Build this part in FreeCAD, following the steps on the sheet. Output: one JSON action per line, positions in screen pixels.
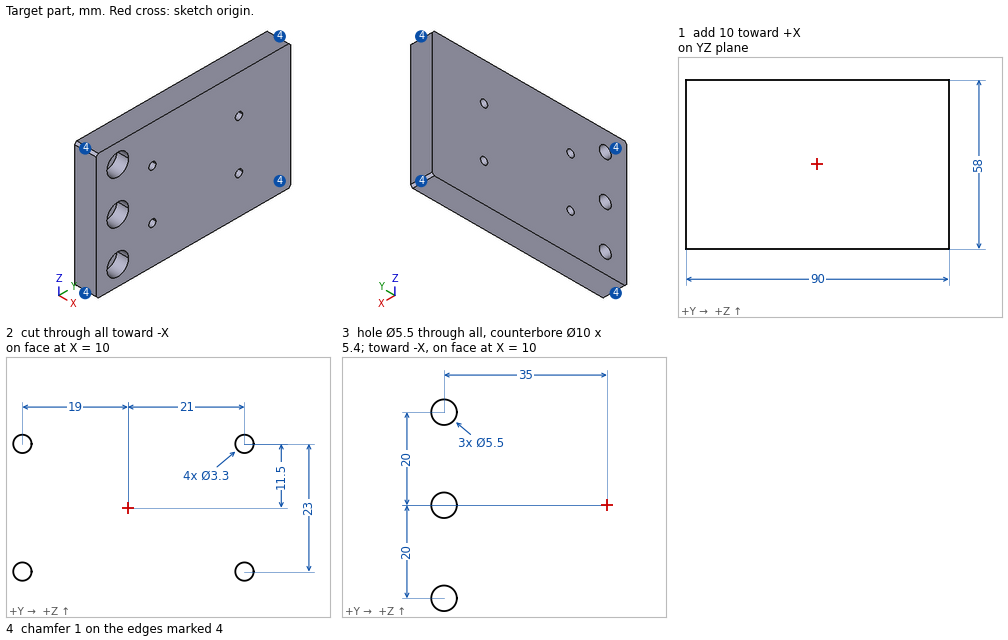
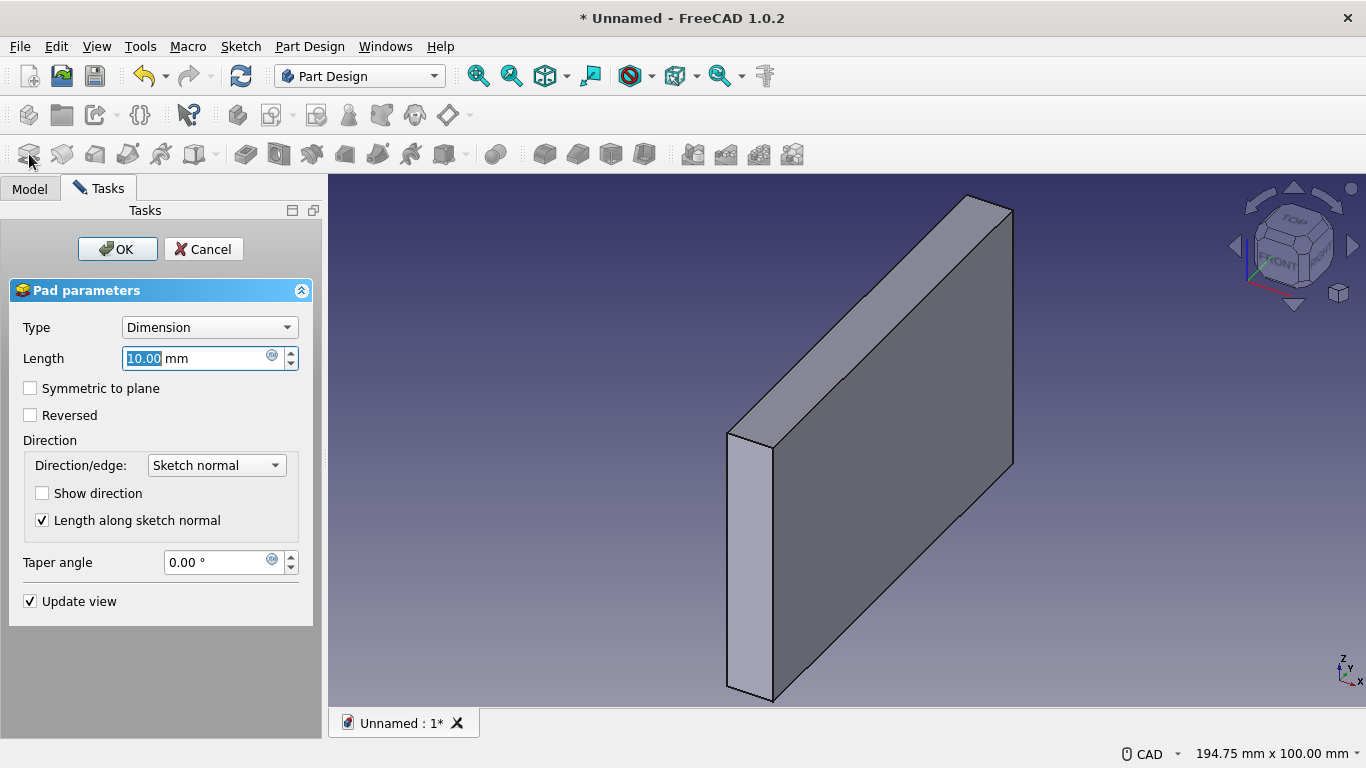
{"action": "type", "text": "10"}
{"action": "key", "text": "Tab"}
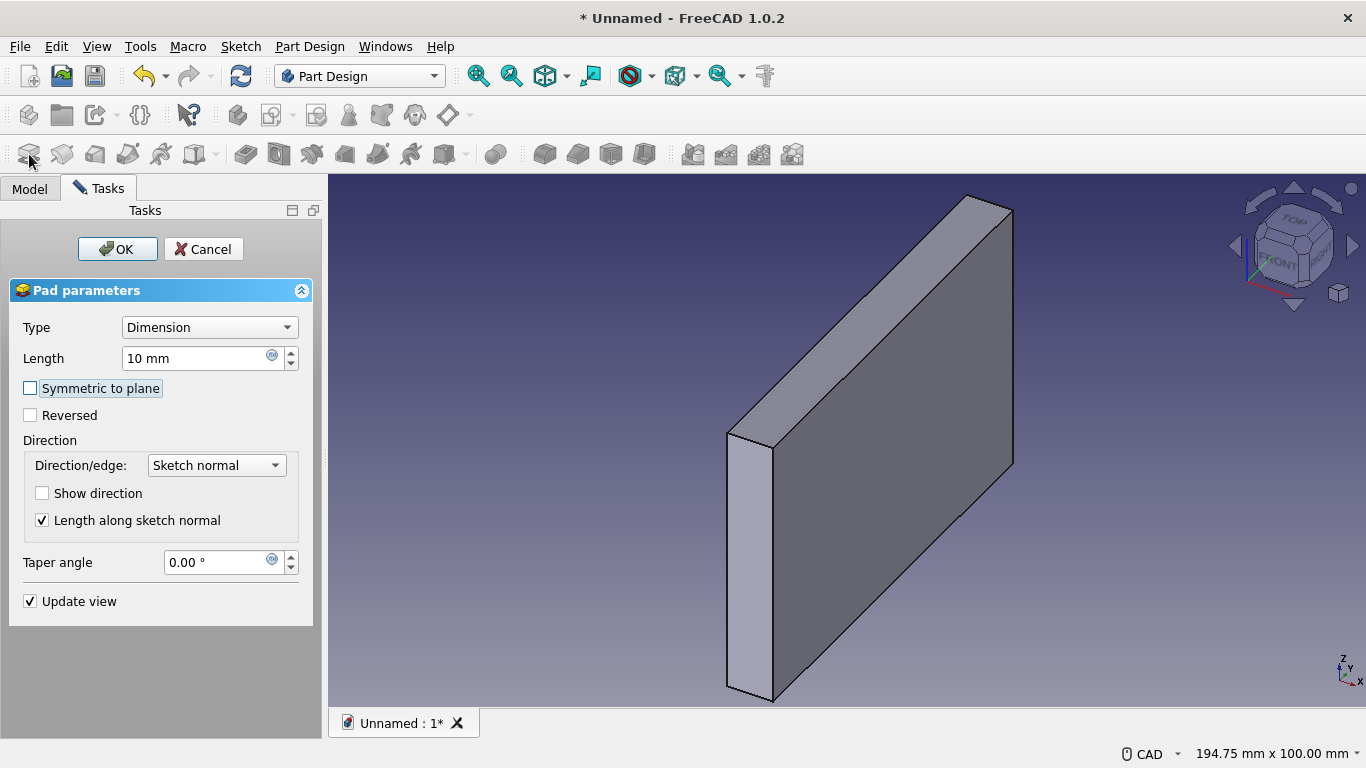
{"action": "left_click", "coordinate": [118, 249]}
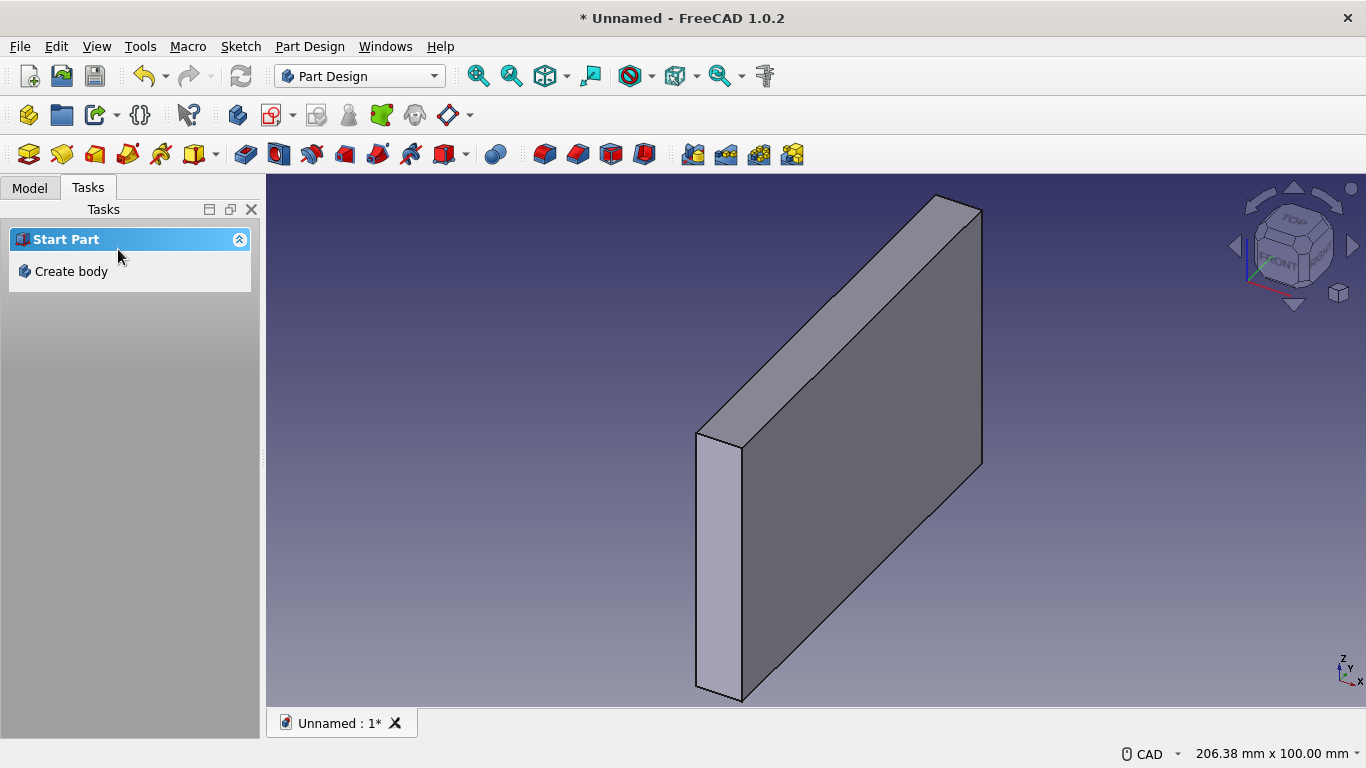
{"action": "left_click", "coordinate": [896, 421]}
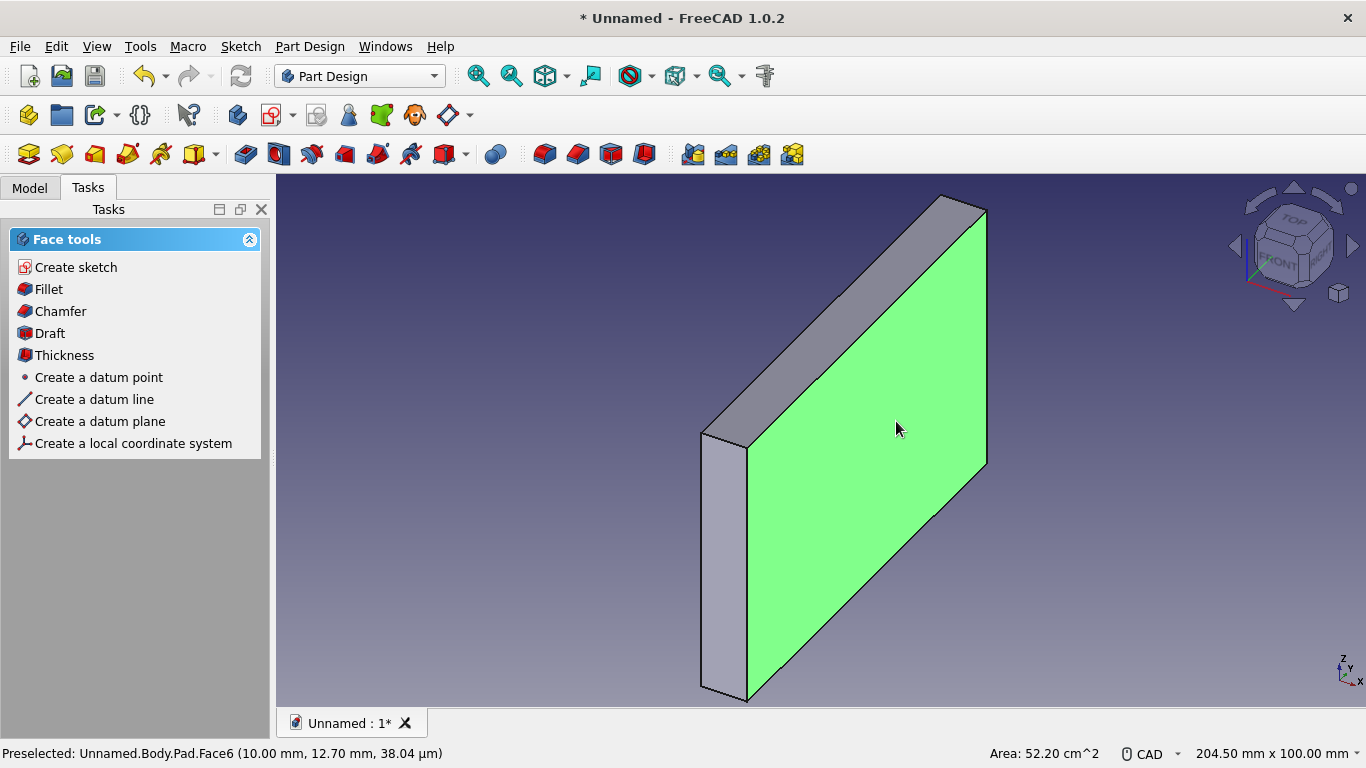
{"action": "left_click", "coordinate": [270, 116]}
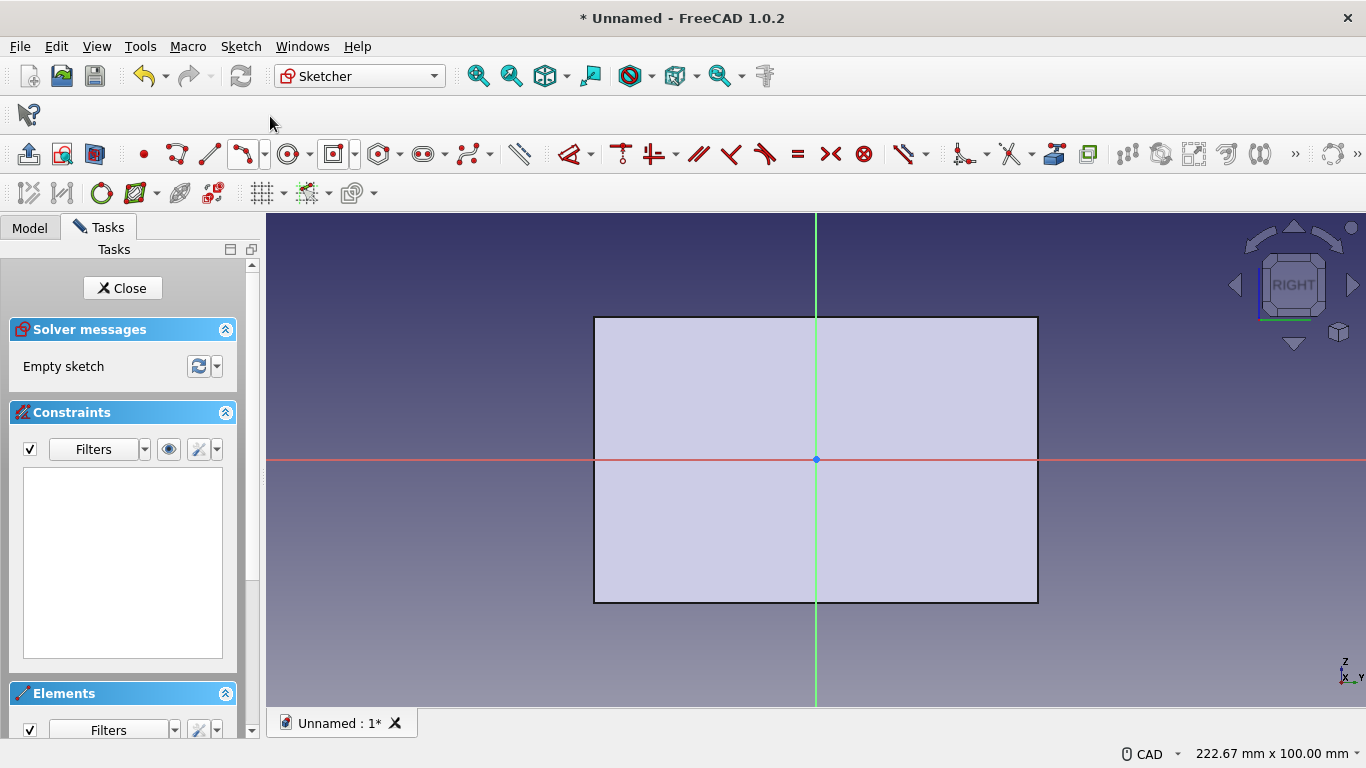
{"action": "scroll", "coordinate": [881, 460], "scroll_direction": "up", "scroll_amount": 4}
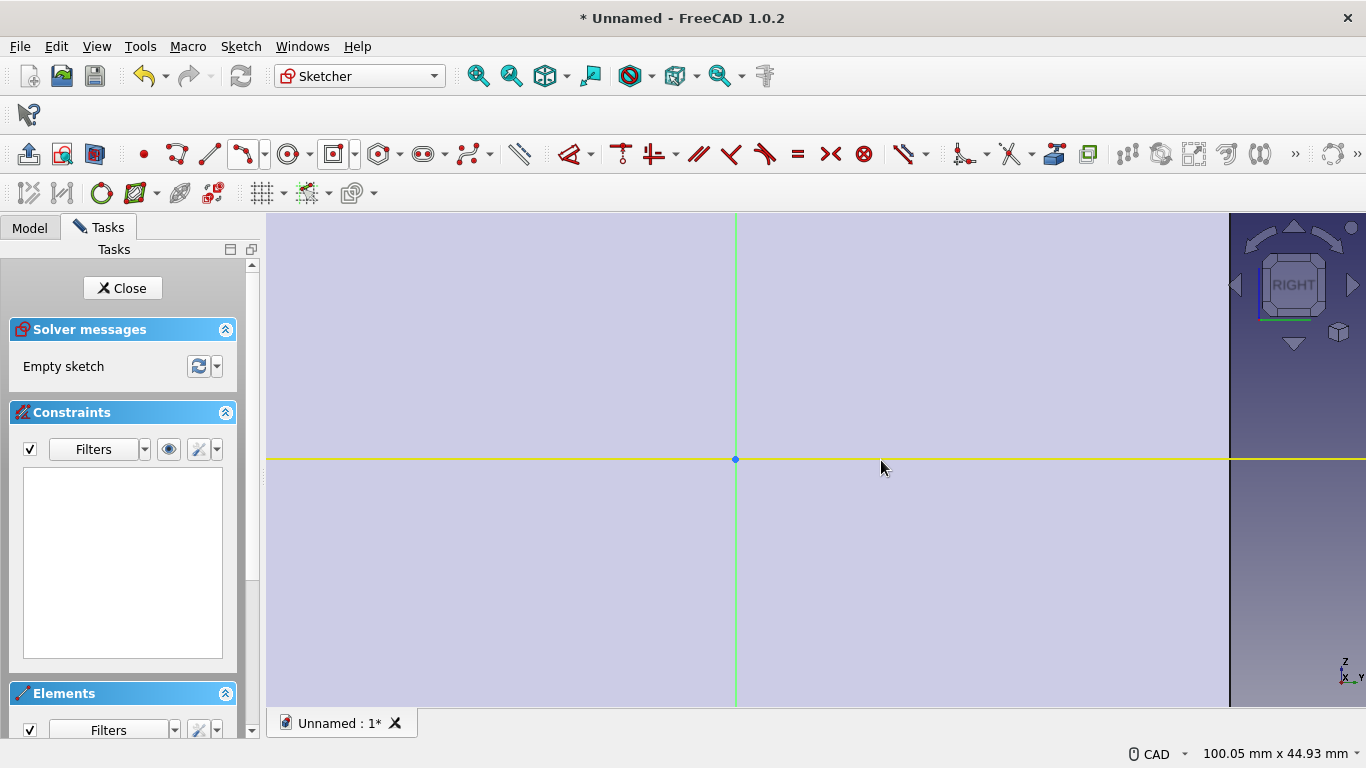
{"action": "left_click", "coordinate": [288, 154]}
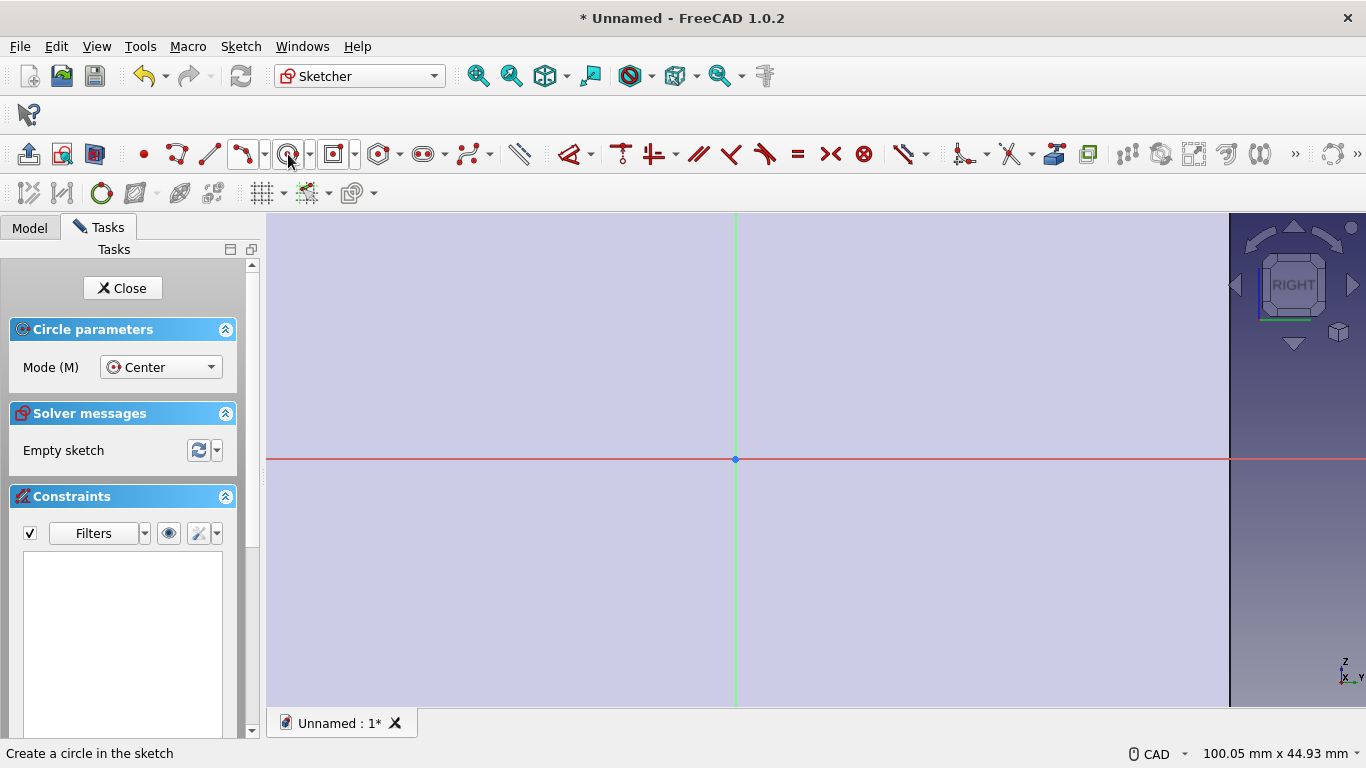
{"action": "scroll", "coordinate": [967, 333], "scroll_direction": "up", "scroll_amount": 2}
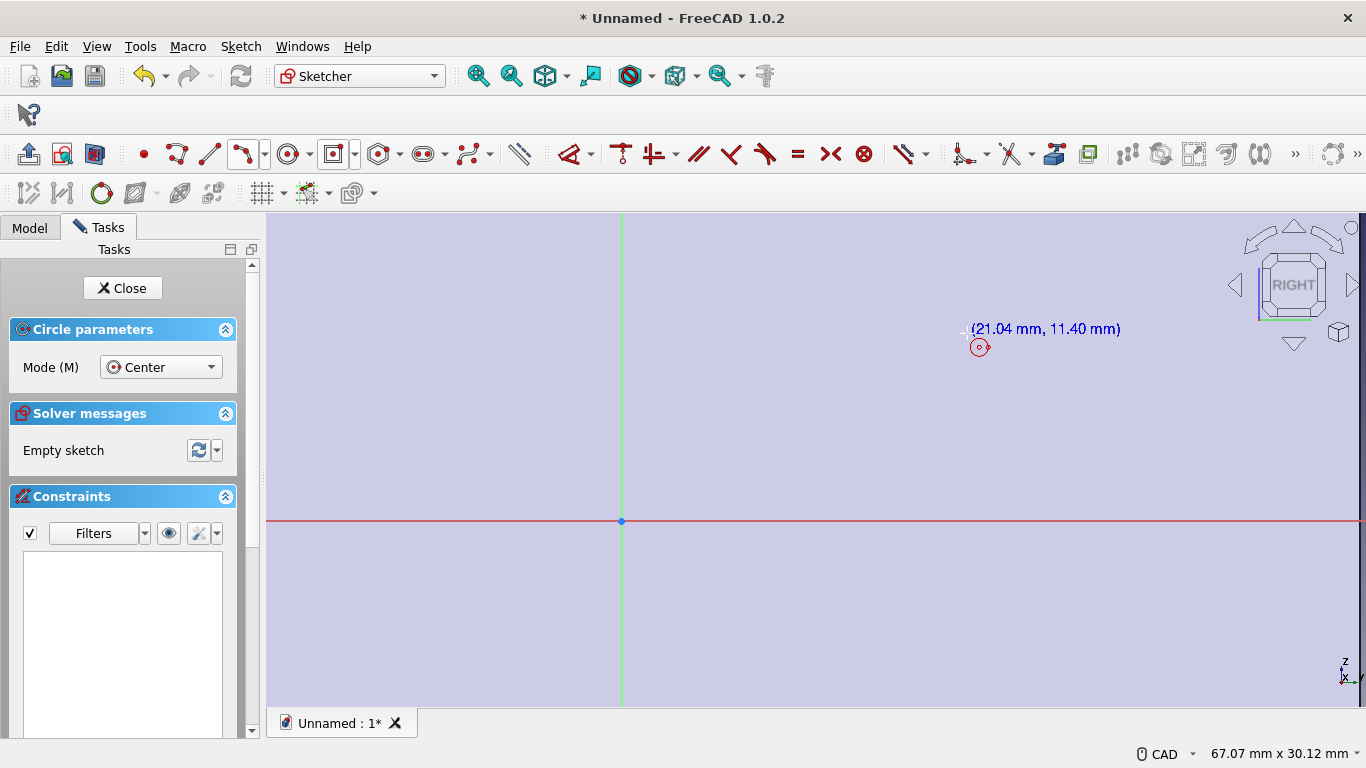
{"action": "left_click", "coordinate": [966, 333]}
{"action": "mouse_move", "coordinate": [985, 314]}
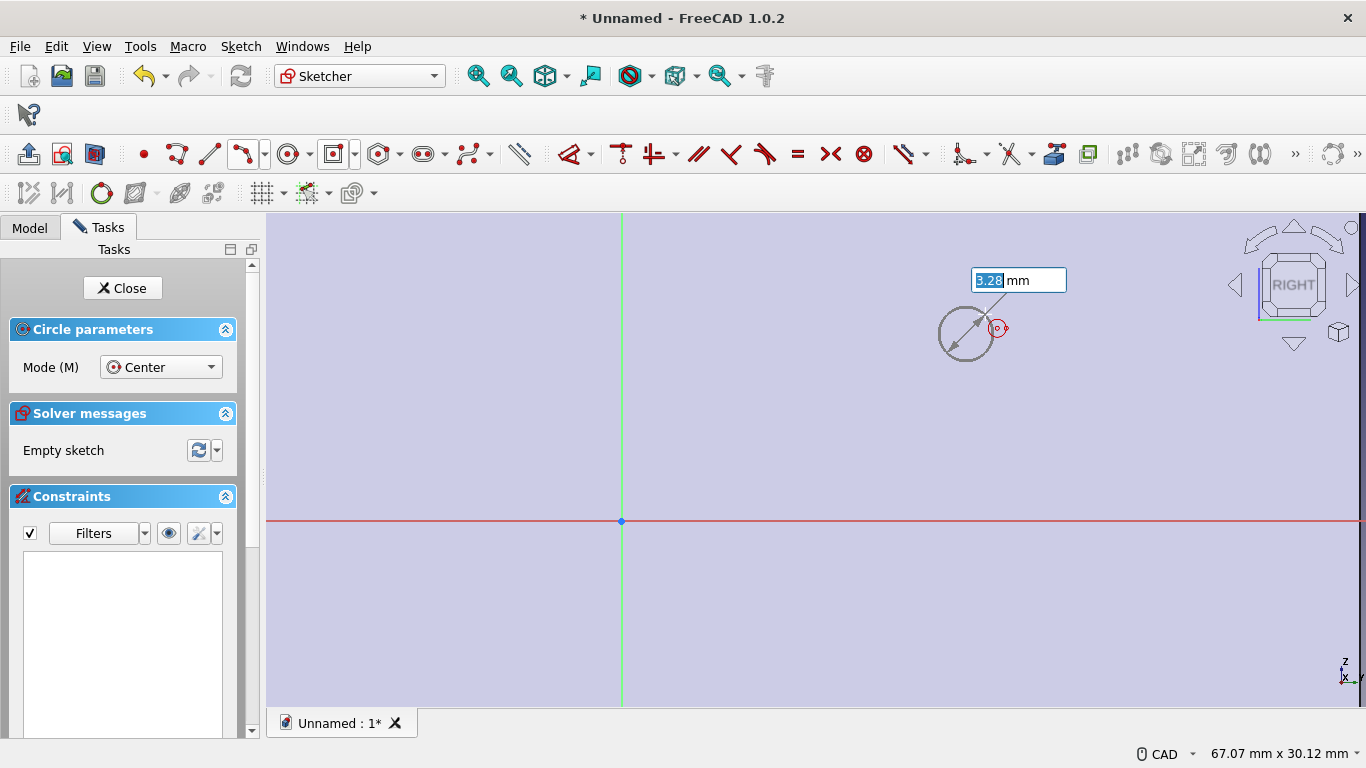
{"action": "type", "text": "3.3"}
{"action": "key", "text": "Return"}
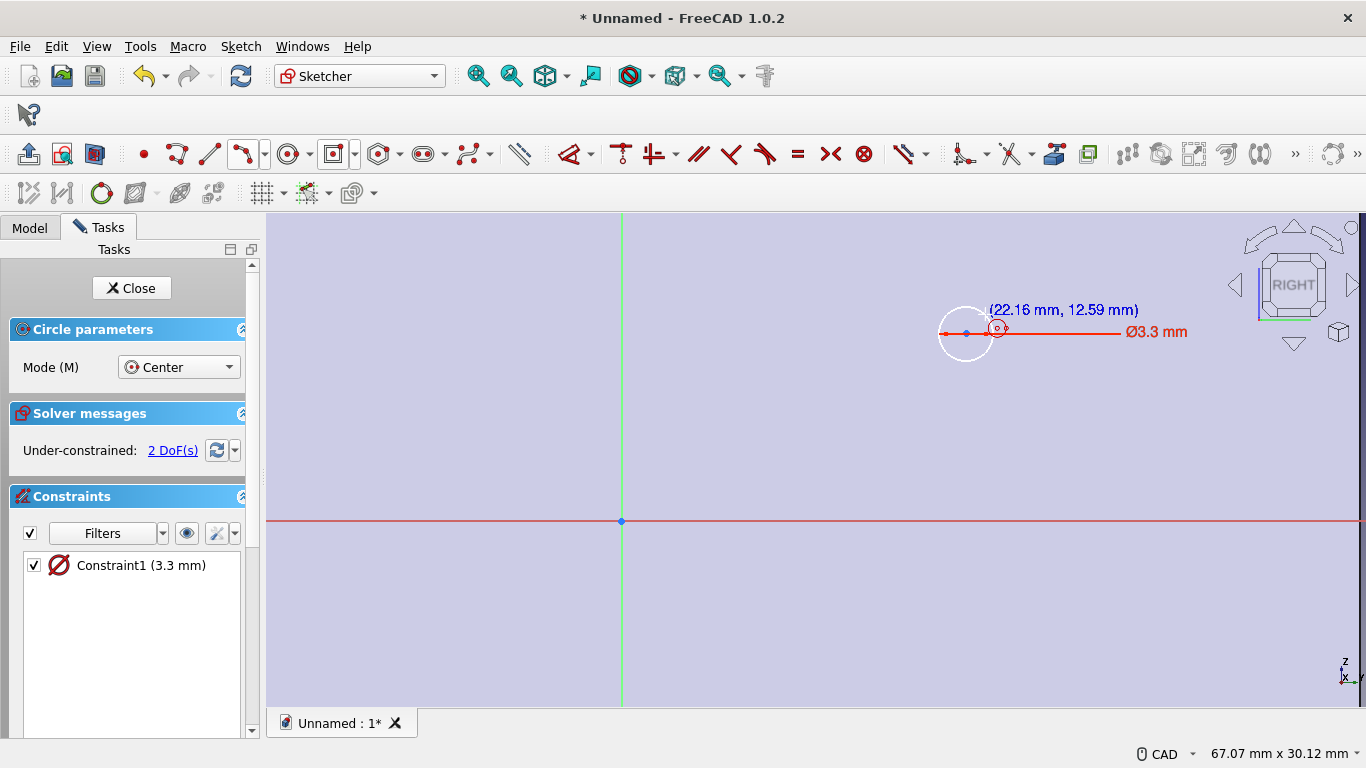
{"action": "scroll", "coordinate": [970, 335], "scroll_direction": "down", "scroll_amount": 2}